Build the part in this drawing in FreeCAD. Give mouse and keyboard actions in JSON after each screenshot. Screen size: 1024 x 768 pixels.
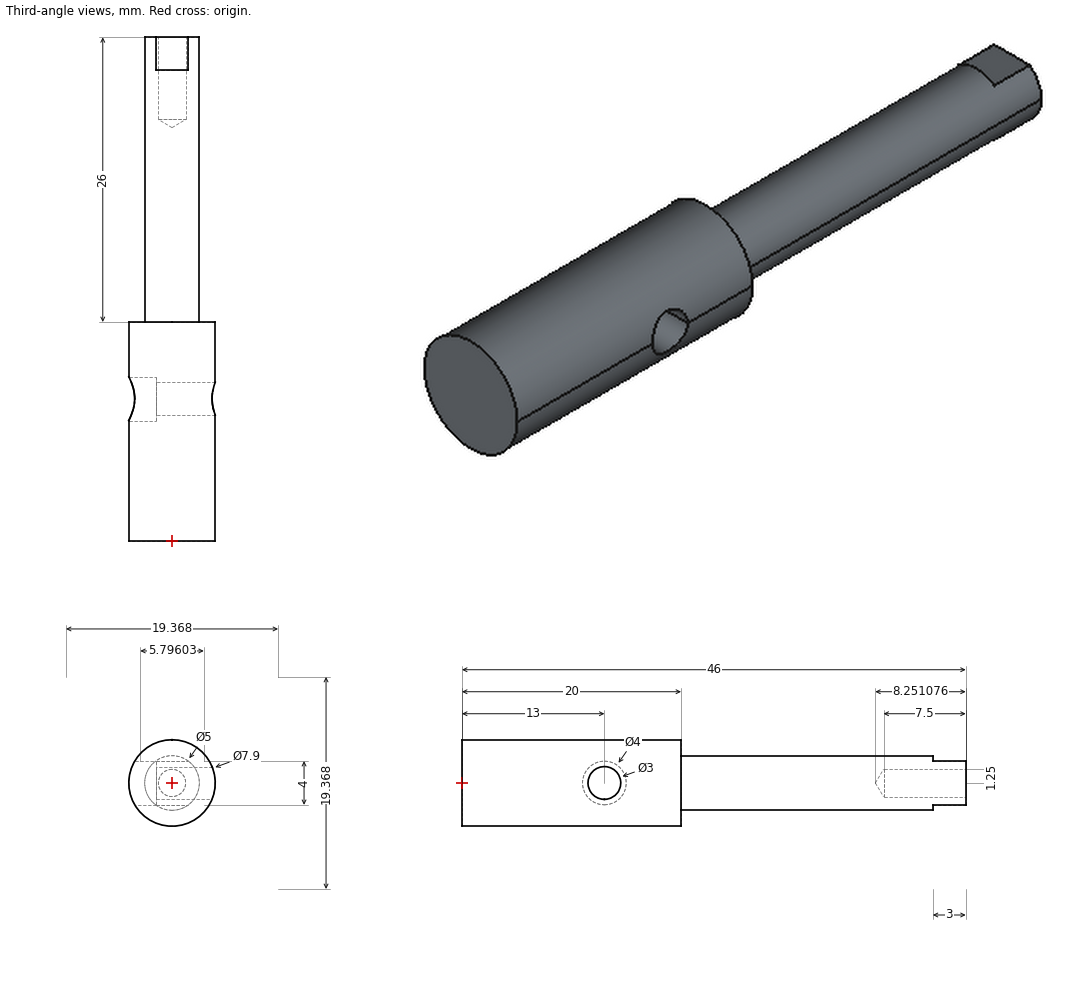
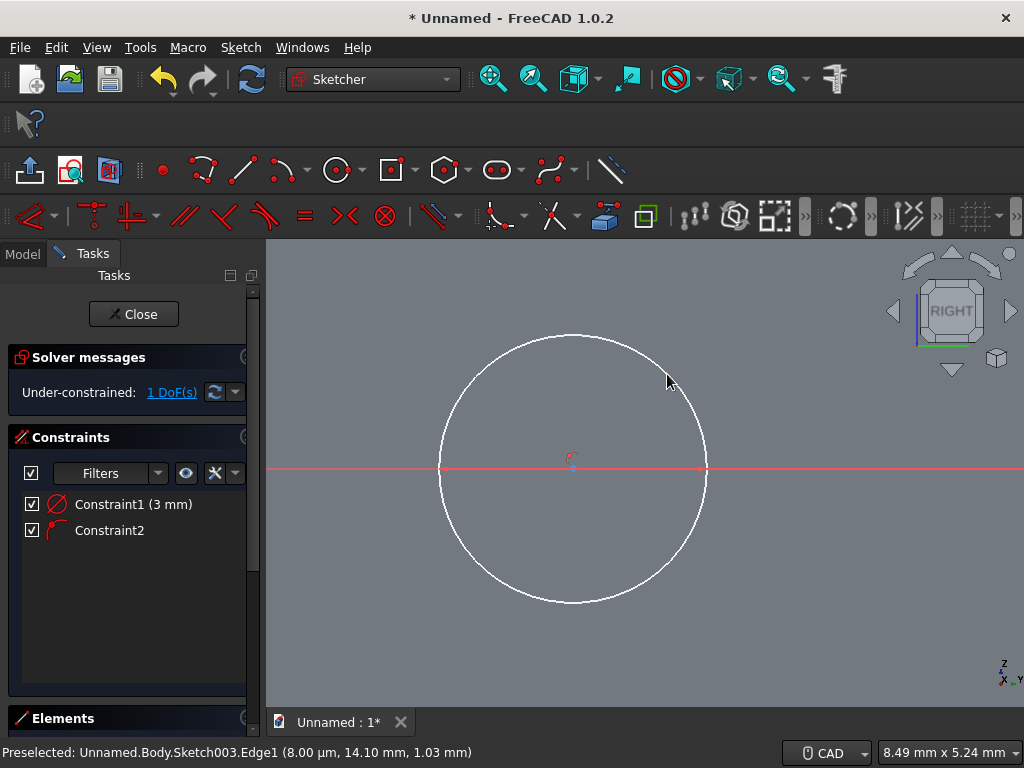
{"action": "left_click", "coordinate": [30, 216]}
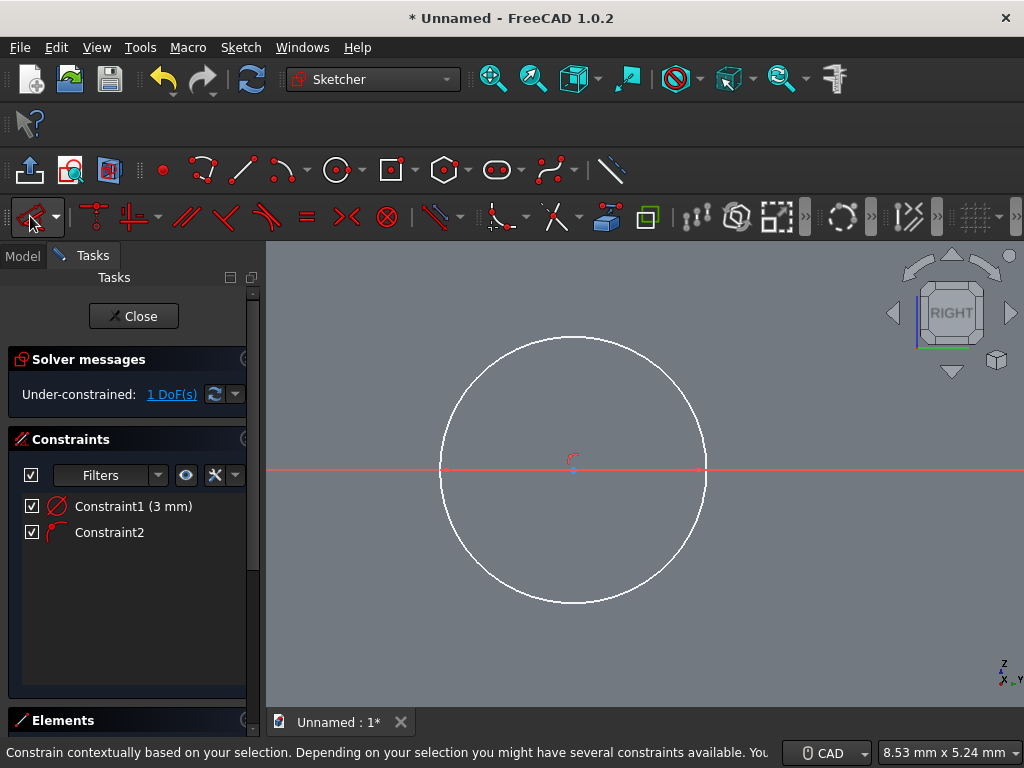
{"action": "left_click", "coordinate": [573, 470]}
{"action": "left_click", "coordinate": [369, 504]}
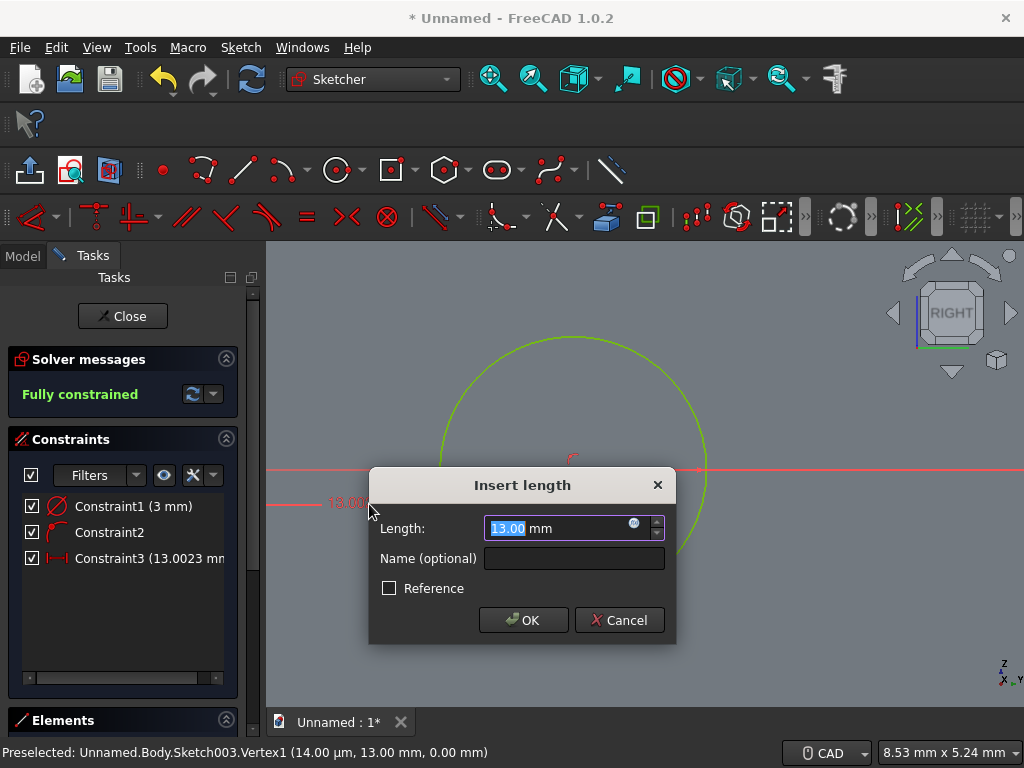
{"action": "type", "text": "13"}
{"action": "key", "text": "Return"}
{"action": "key", "text": "Escape"}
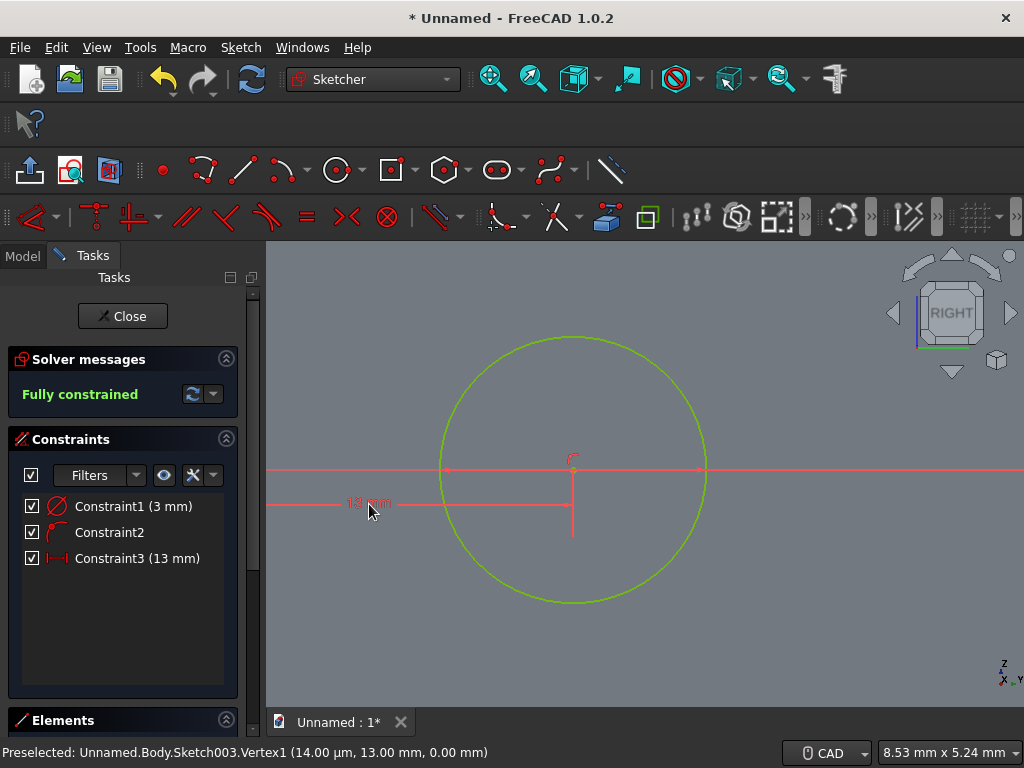
{"action": "left_click", "coordinate": [123, 316]}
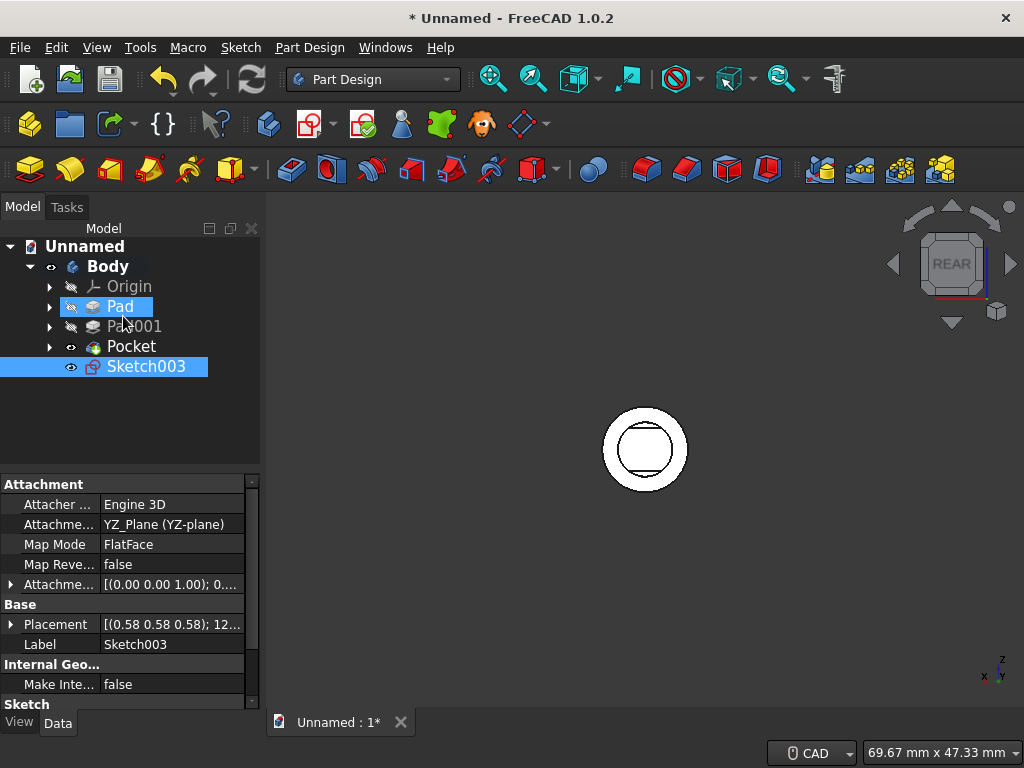
{"action": "left_click", "coordinate": [292, 170]}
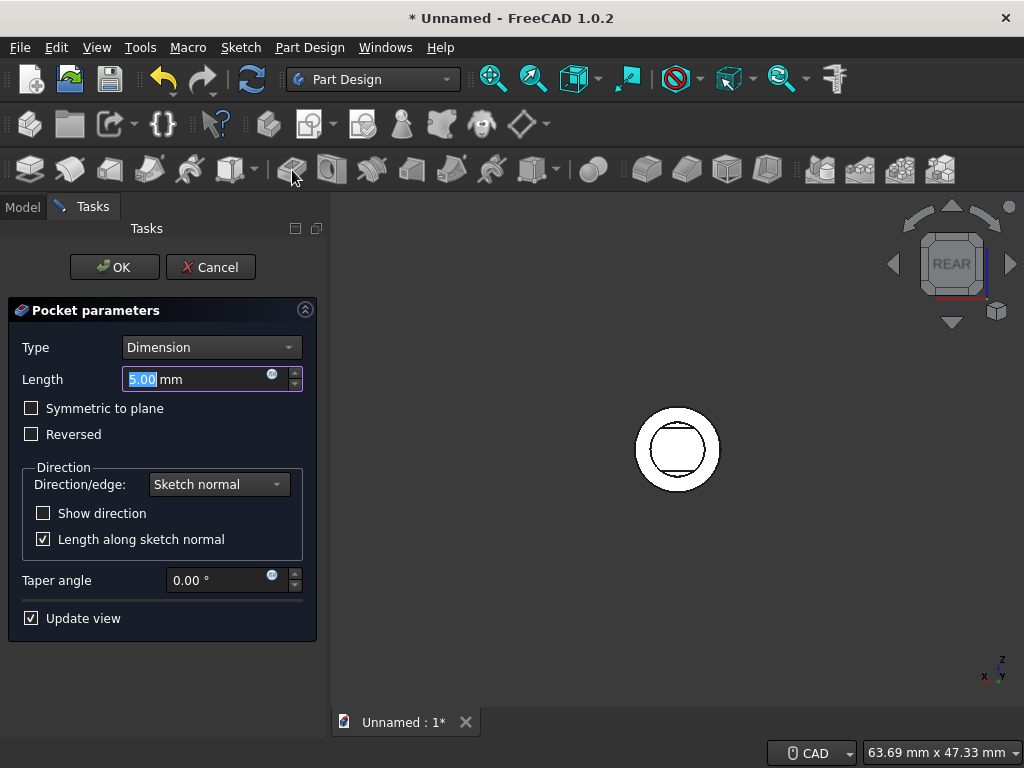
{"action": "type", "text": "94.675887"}
{"action": "key", "text": "Tab"}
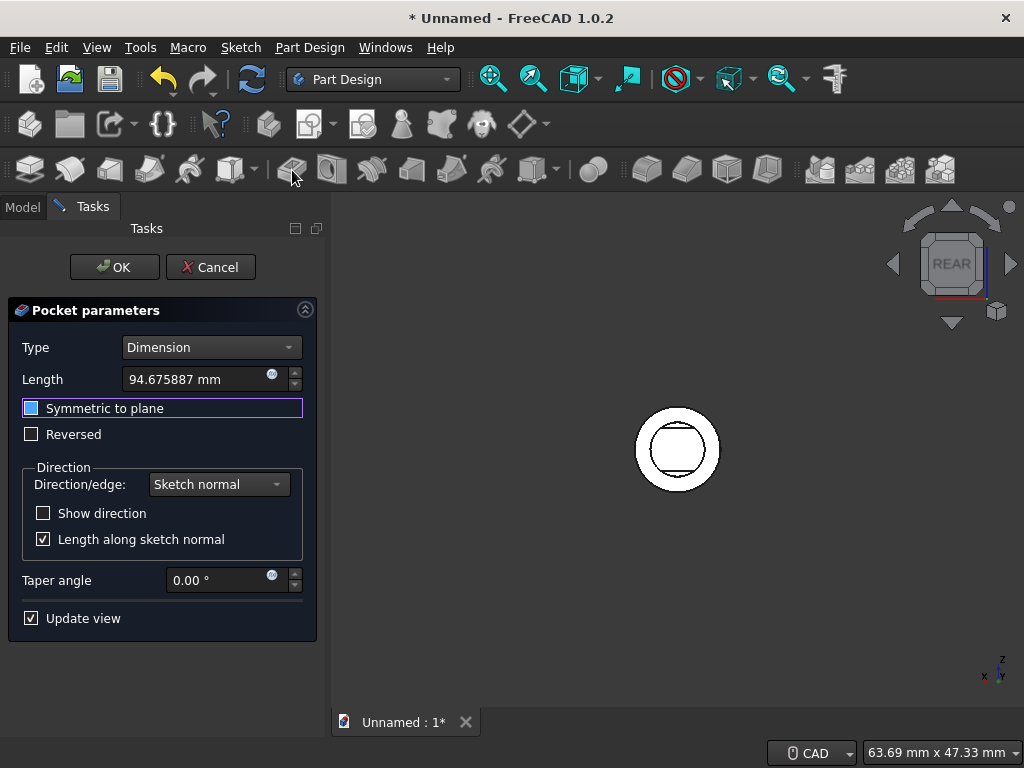
{"action": "left_click", "coordinate": [30, 408]}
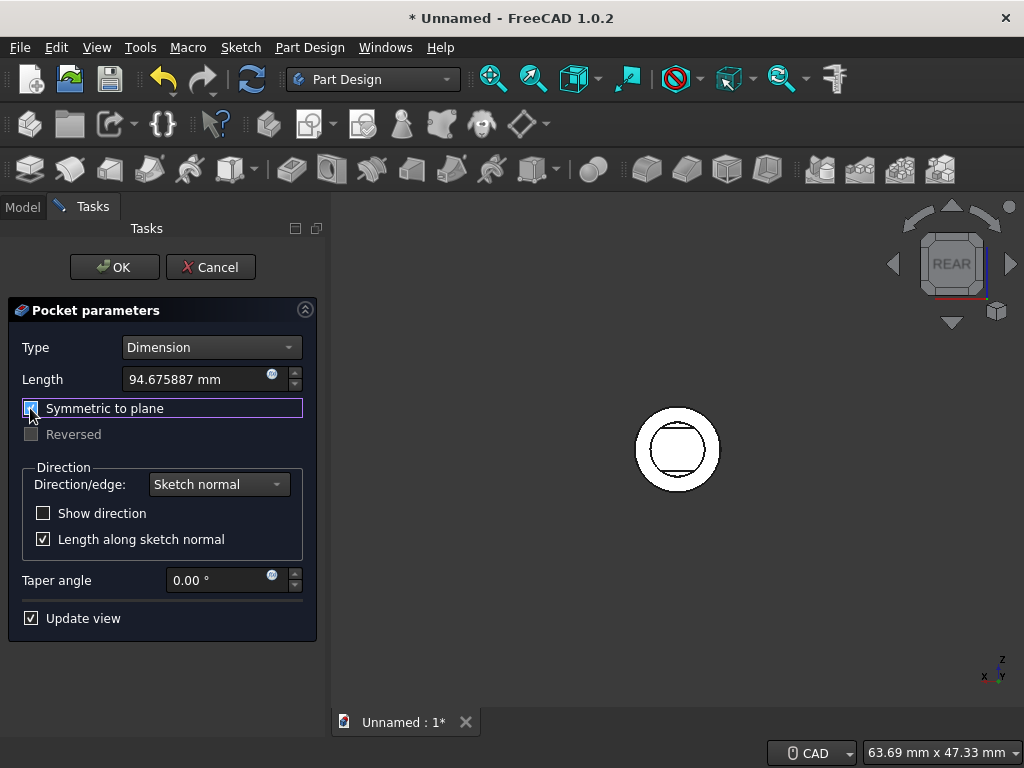
{"action": "left_click", "coordinate": [115, 267]}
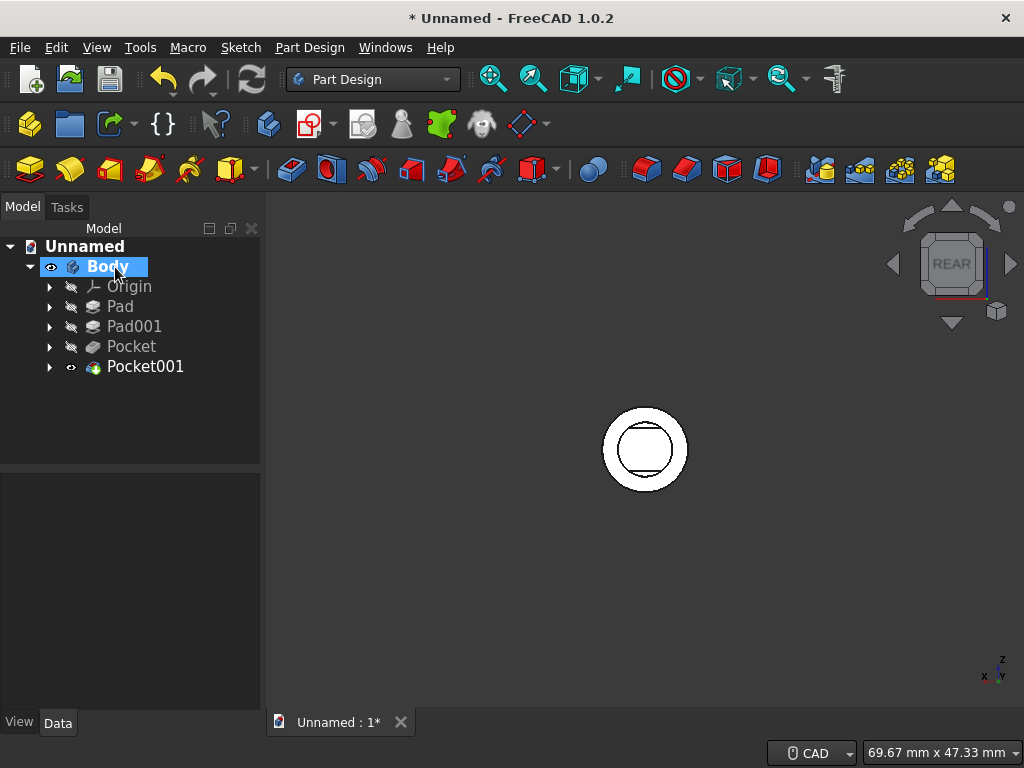
{"action": "left_click", "coordinate": [494, 80]}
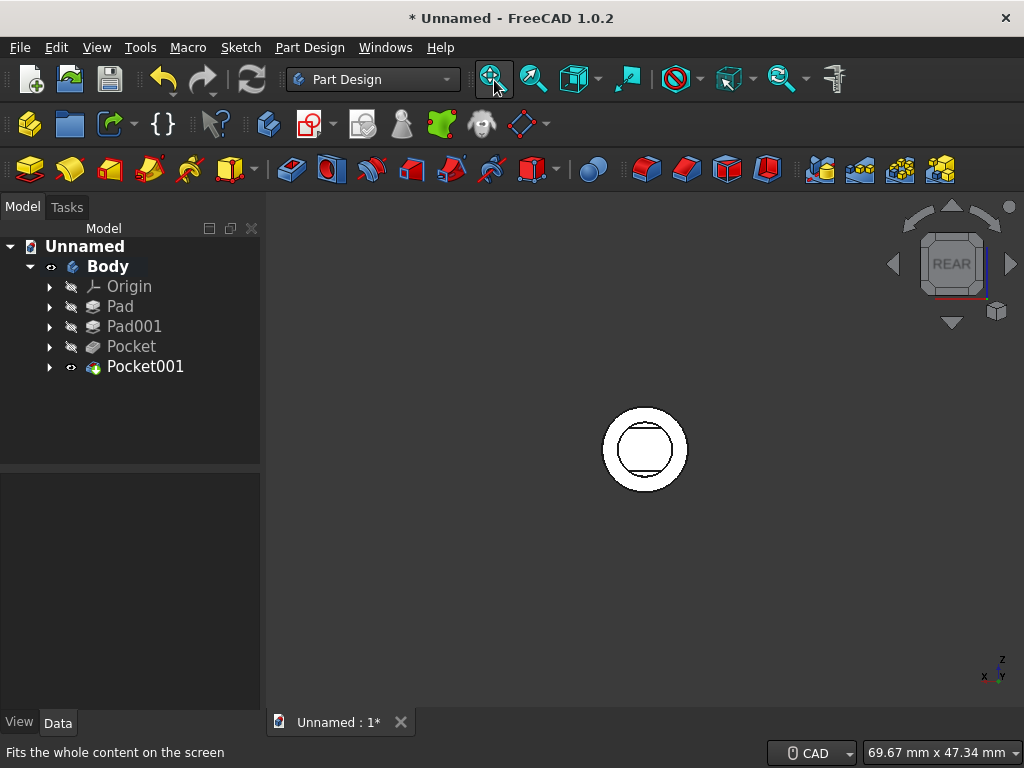
{"action": "left_click", "coordinate": [50, 287]}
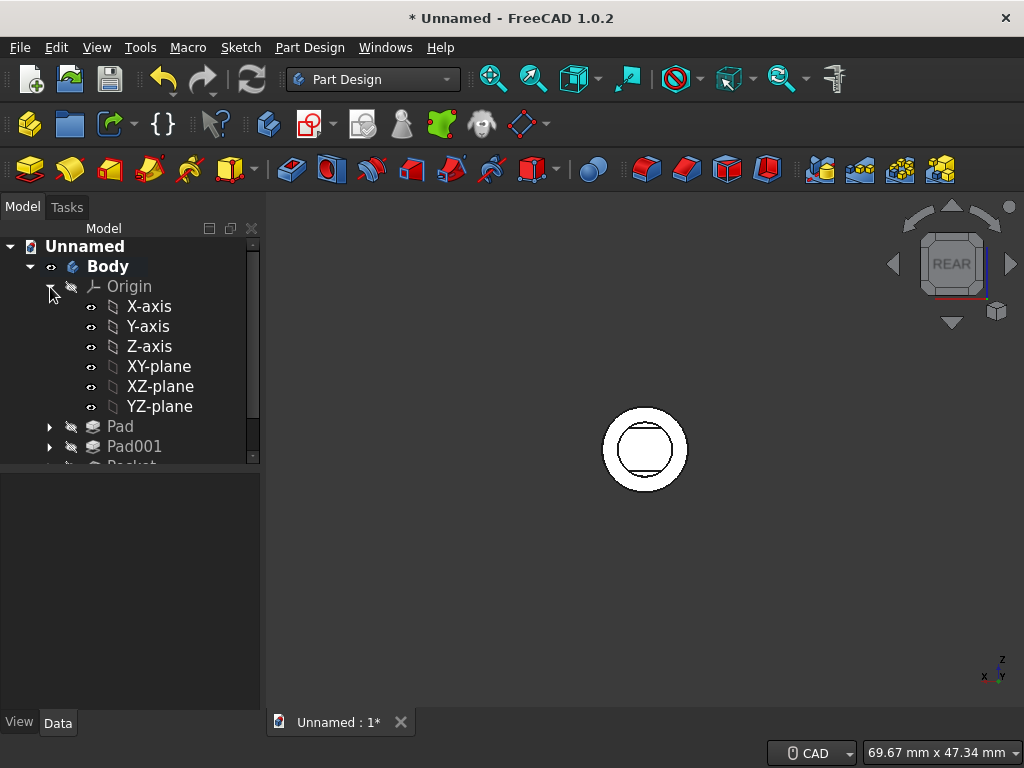
{"action": "left_click", "coordinate": [136, 407]}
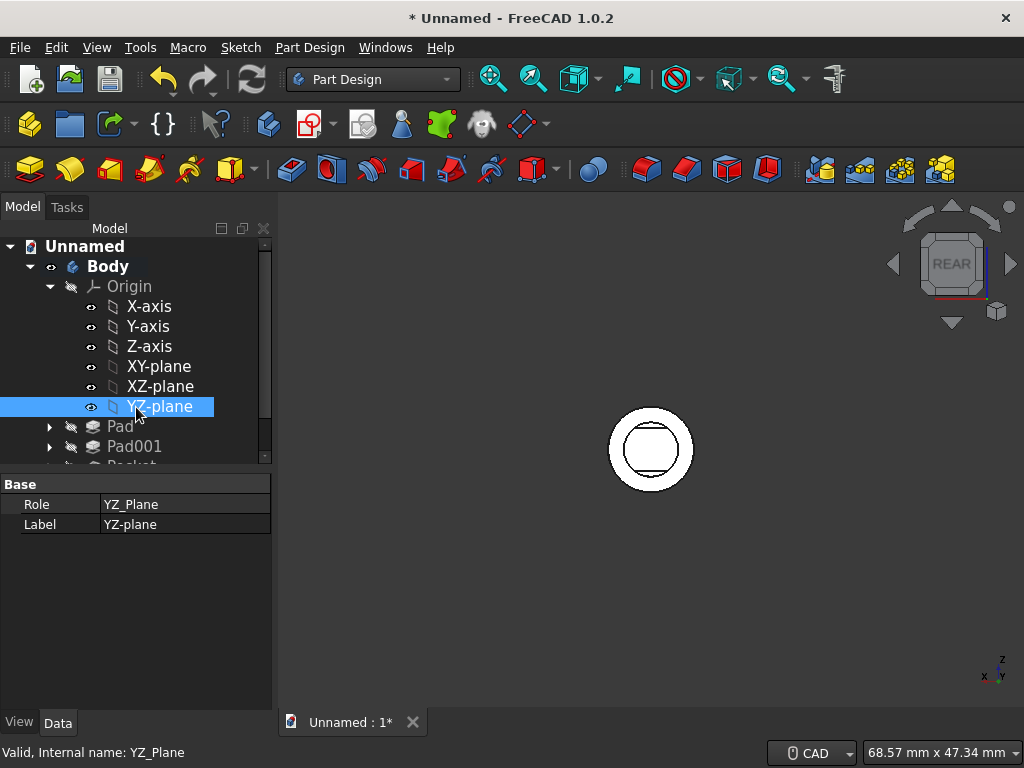
{"action": "left_click", "coordinate": [522, 124]}